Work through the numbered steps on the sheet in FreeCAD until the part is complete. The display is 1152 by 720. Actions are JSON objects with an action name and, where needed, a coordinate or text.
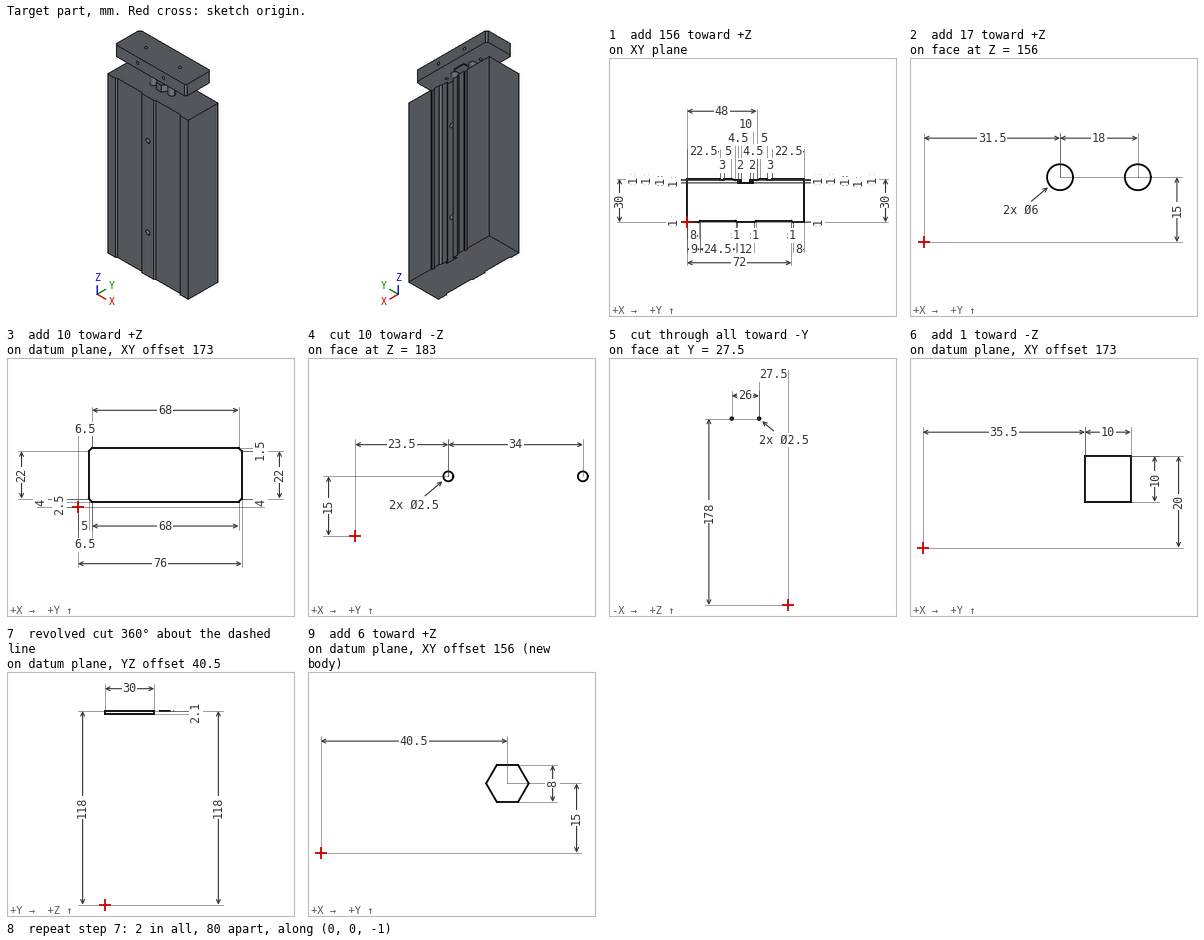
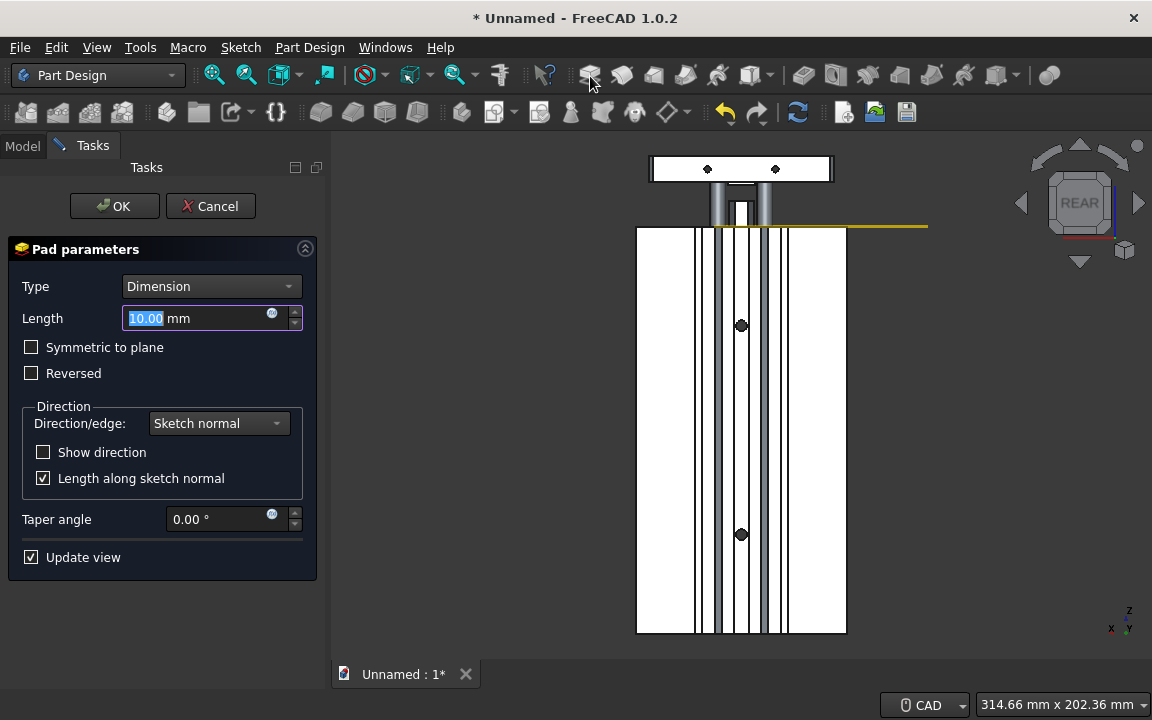
{"action": "type", "text": "6"}
{"action": "key", "text": "Tab"}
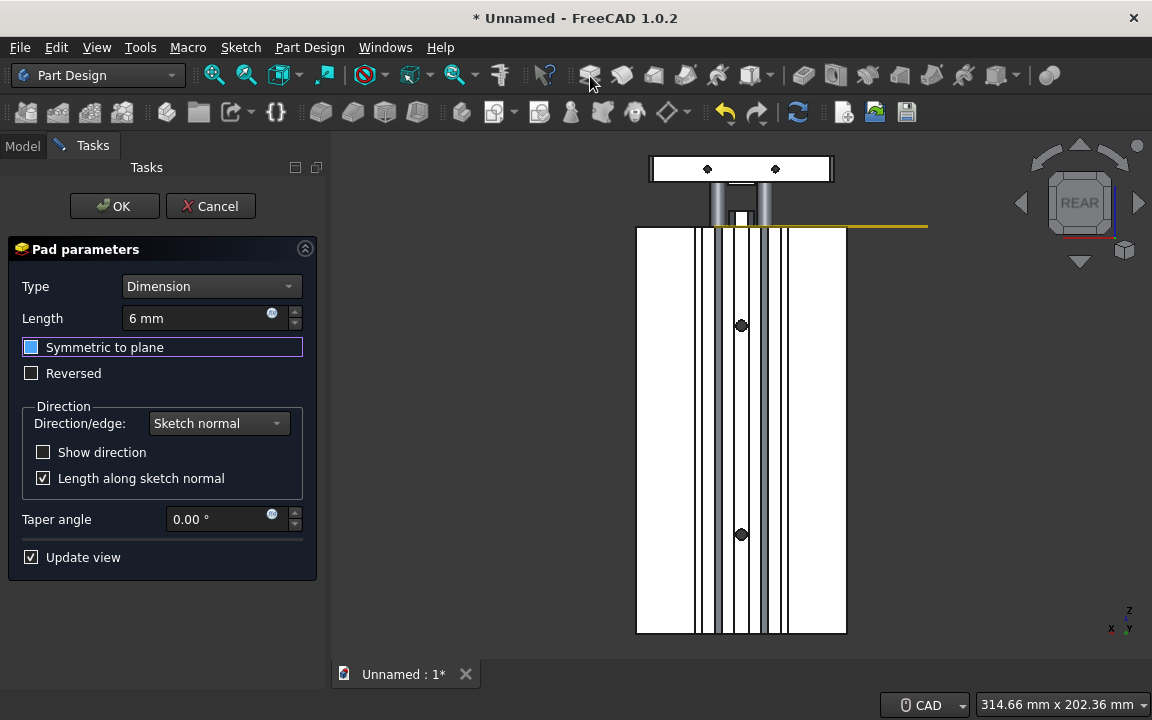
{"action": "left_click", "coordinate": [115, 206]}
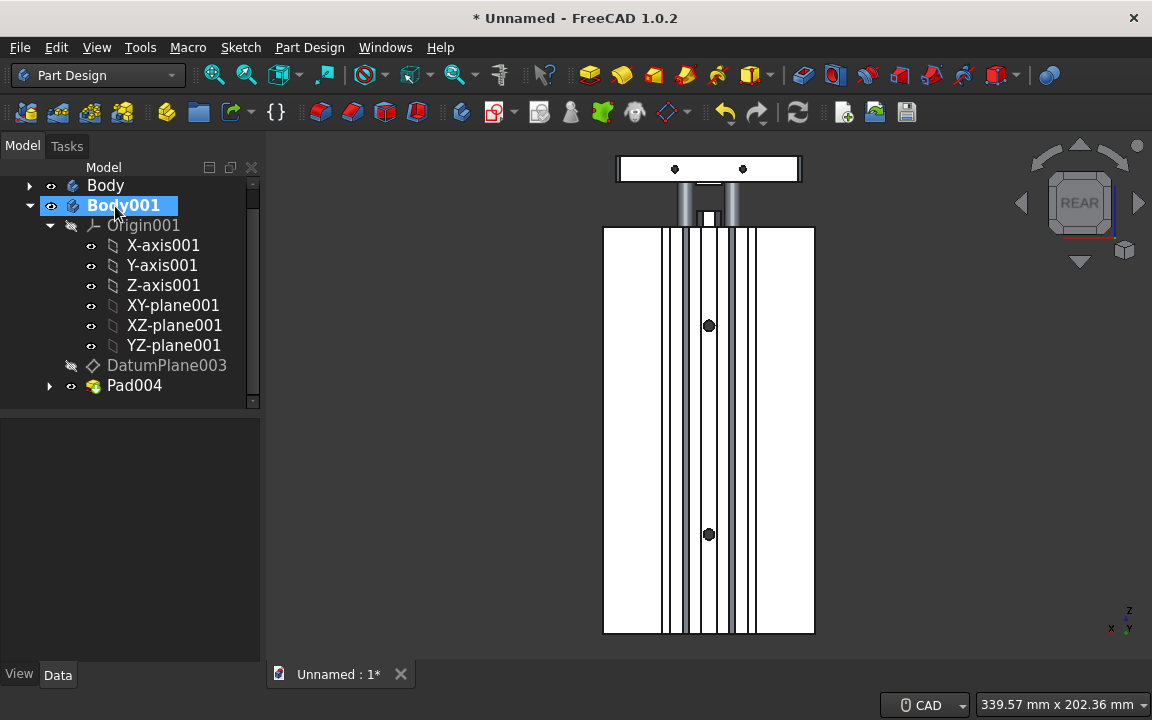
{"action": "key", "text": "0"}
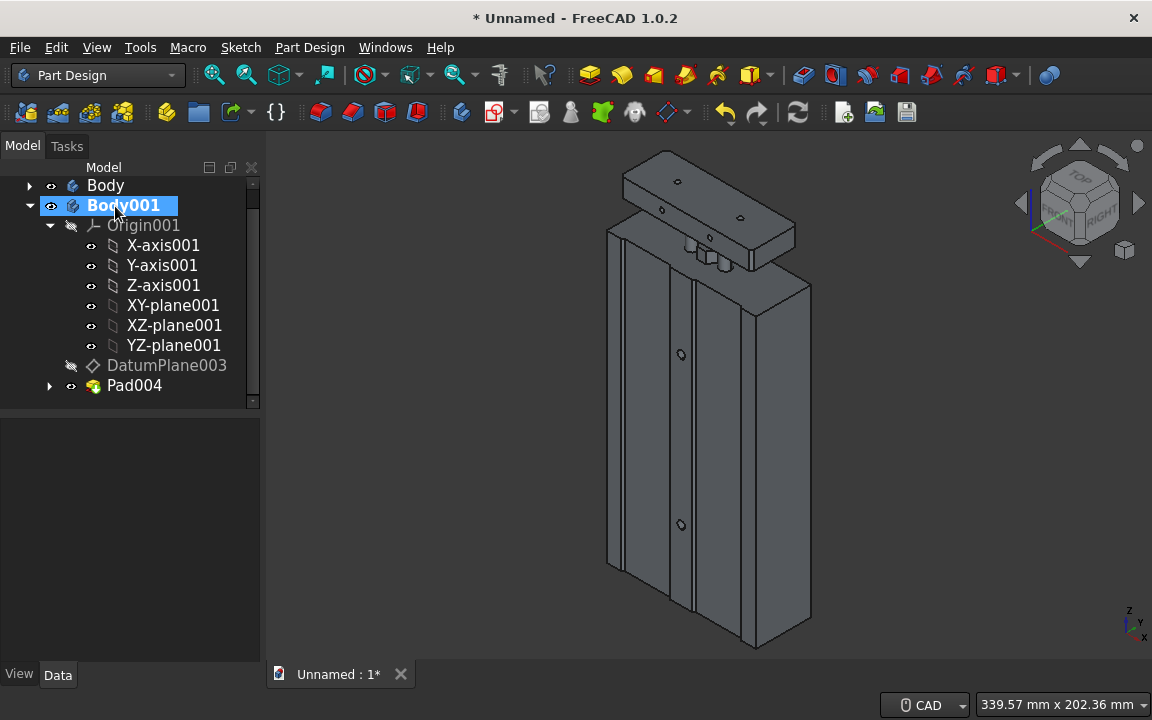
{"action": "key", "text": "v f"}